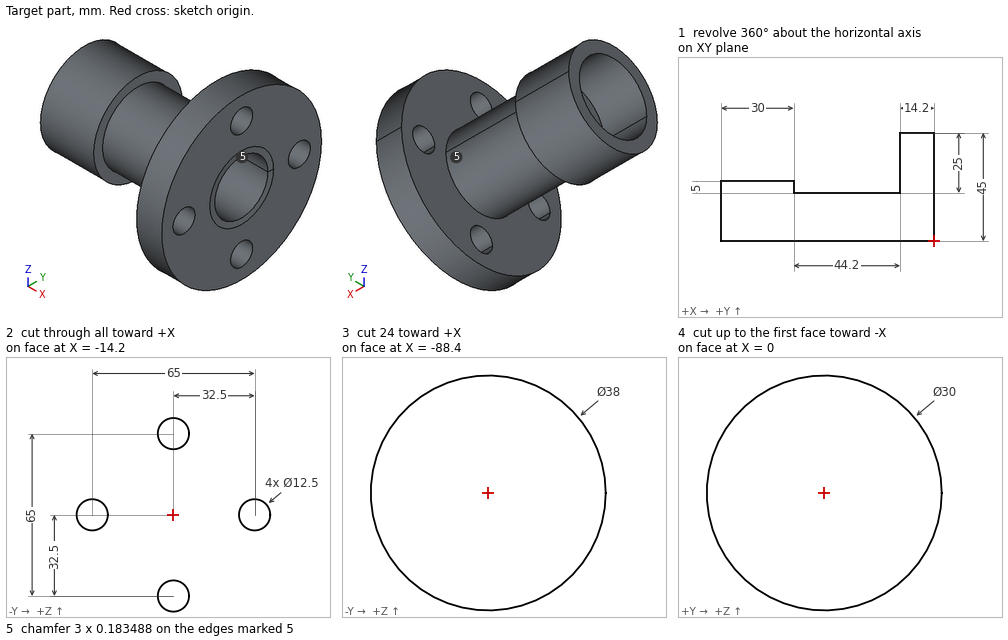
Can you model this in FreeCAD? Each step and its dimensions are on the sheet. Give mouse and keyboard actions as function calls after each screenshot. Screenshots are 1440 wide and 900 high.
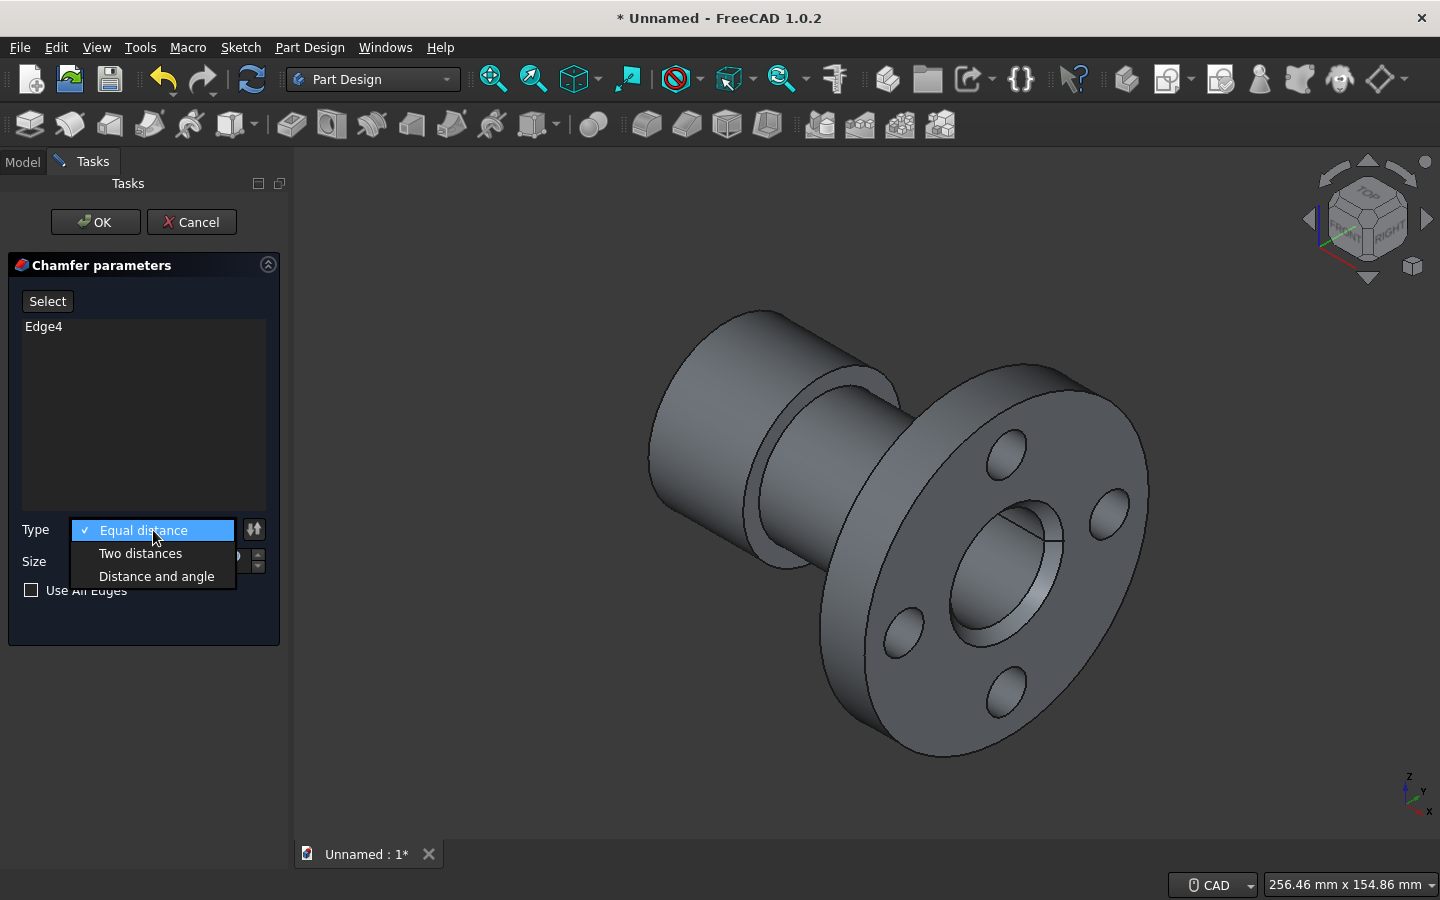
click(152, 554)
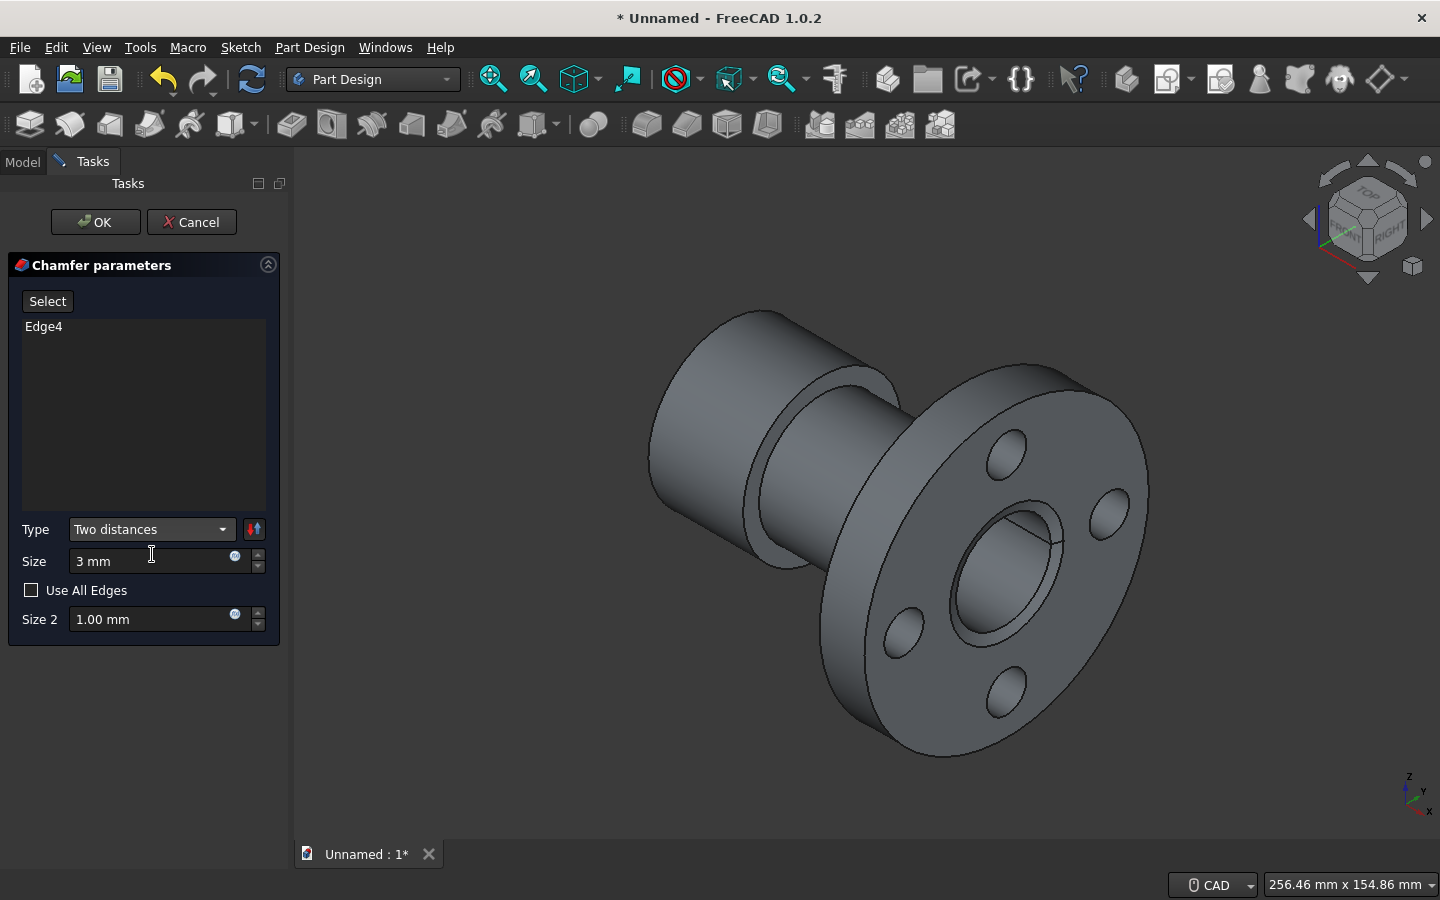
triple_click(160, 619)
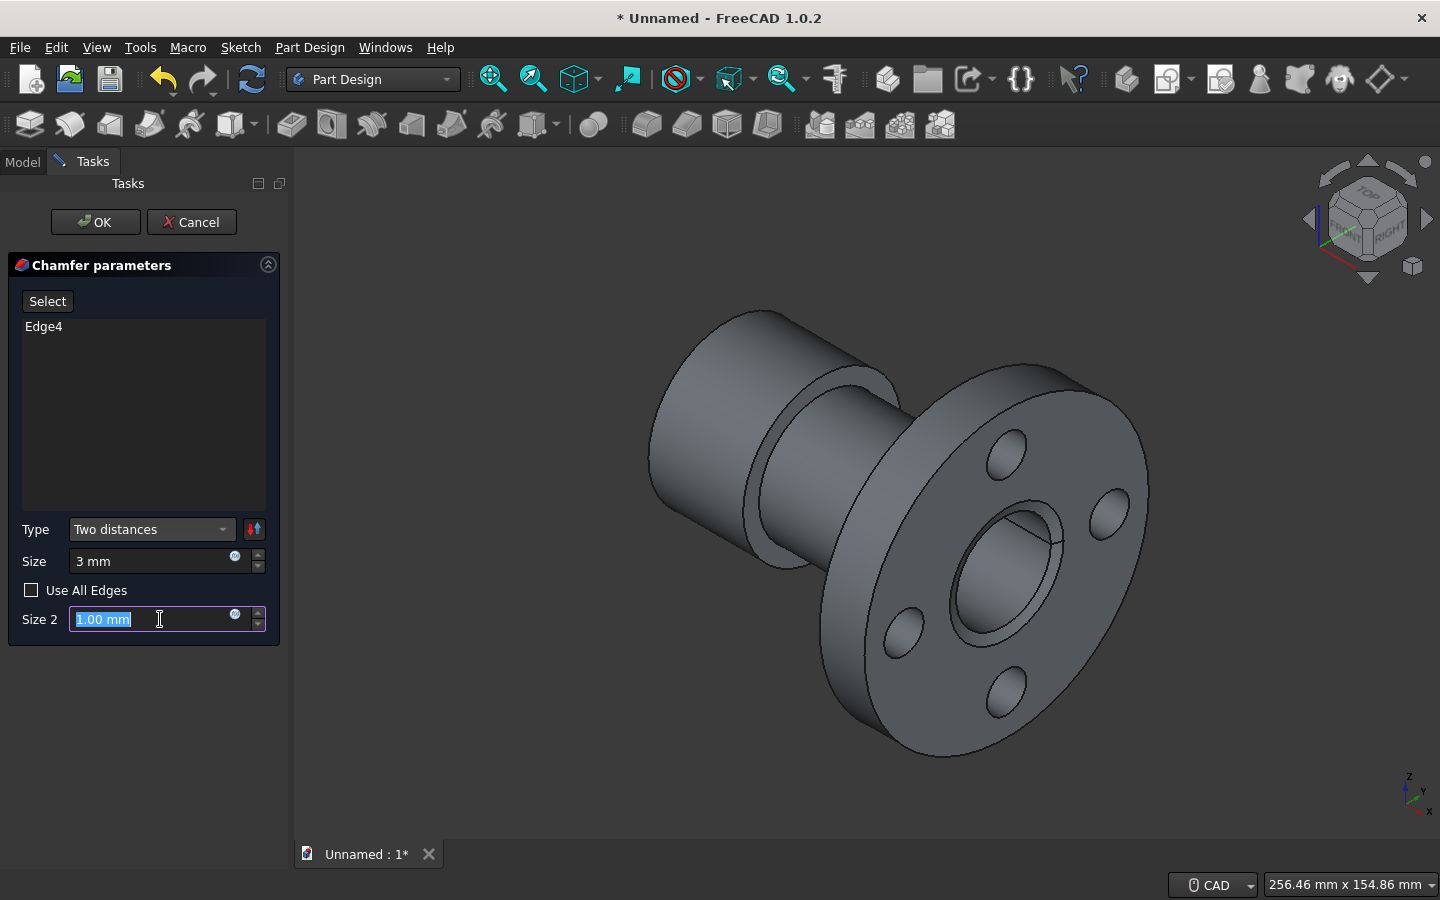
text(0.183488)
key(Tab)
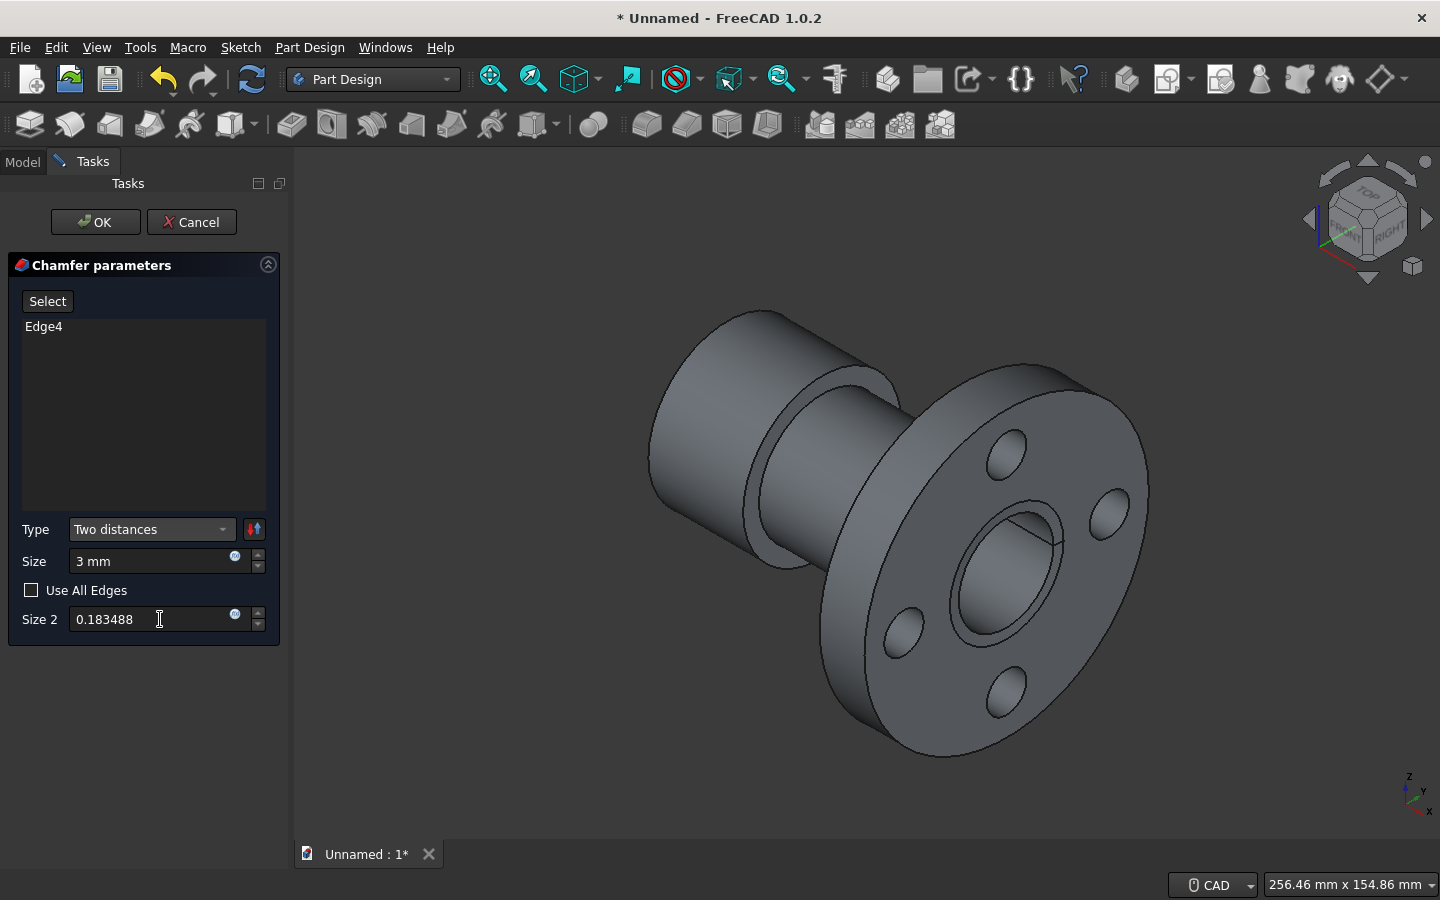
click(96, 222)